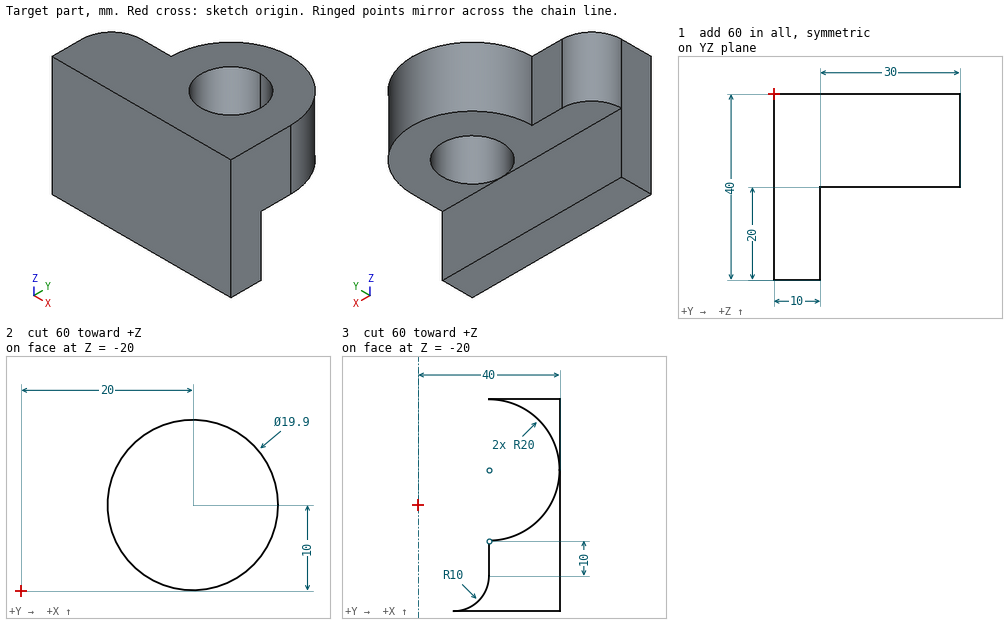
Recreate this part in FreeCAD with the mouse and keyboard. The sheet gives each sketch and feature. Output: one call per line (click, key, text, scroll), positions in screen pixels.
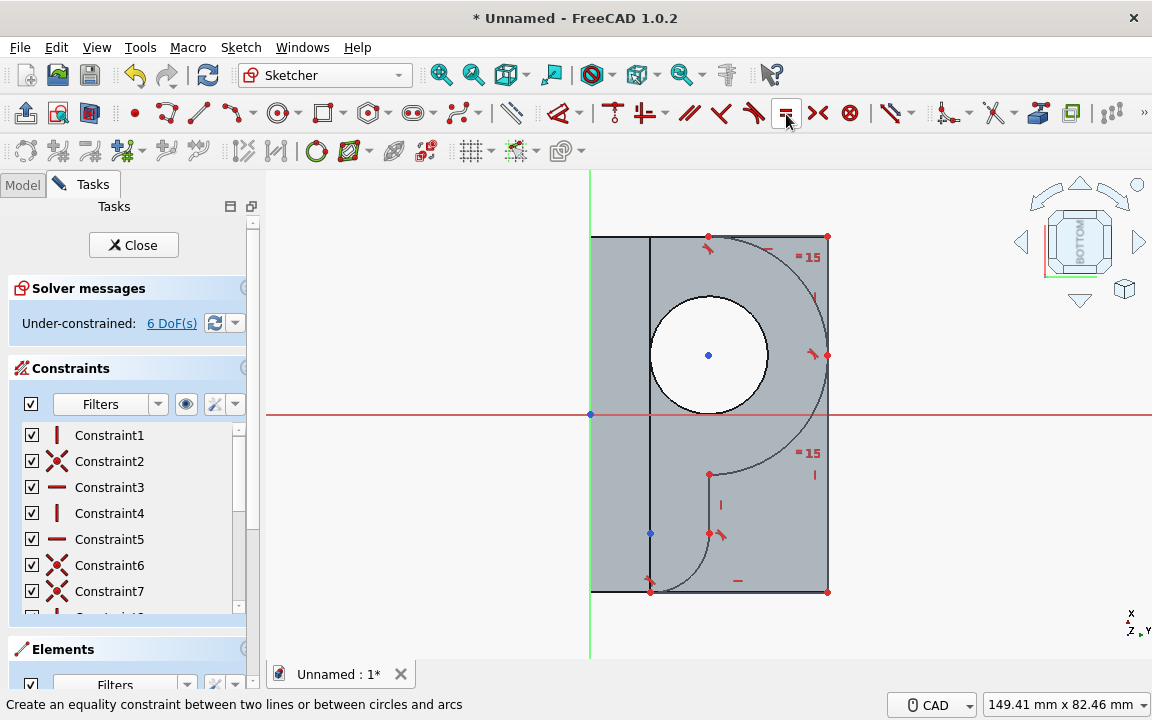
click(709, 356)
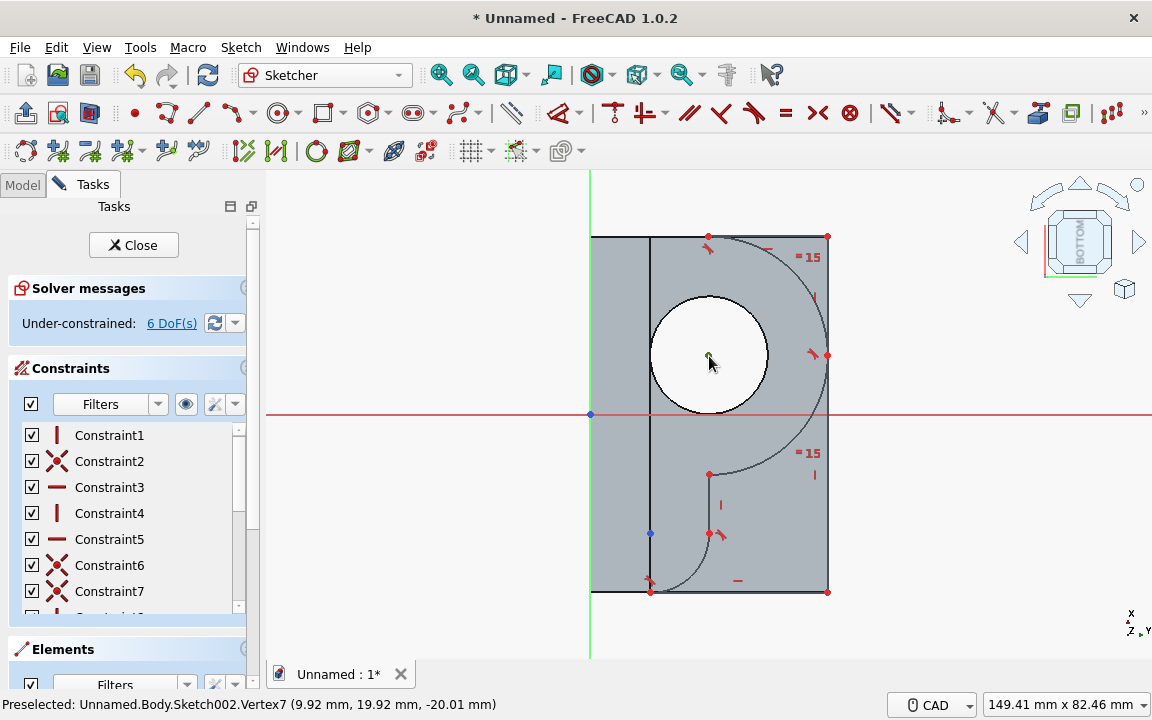
click(709, 475)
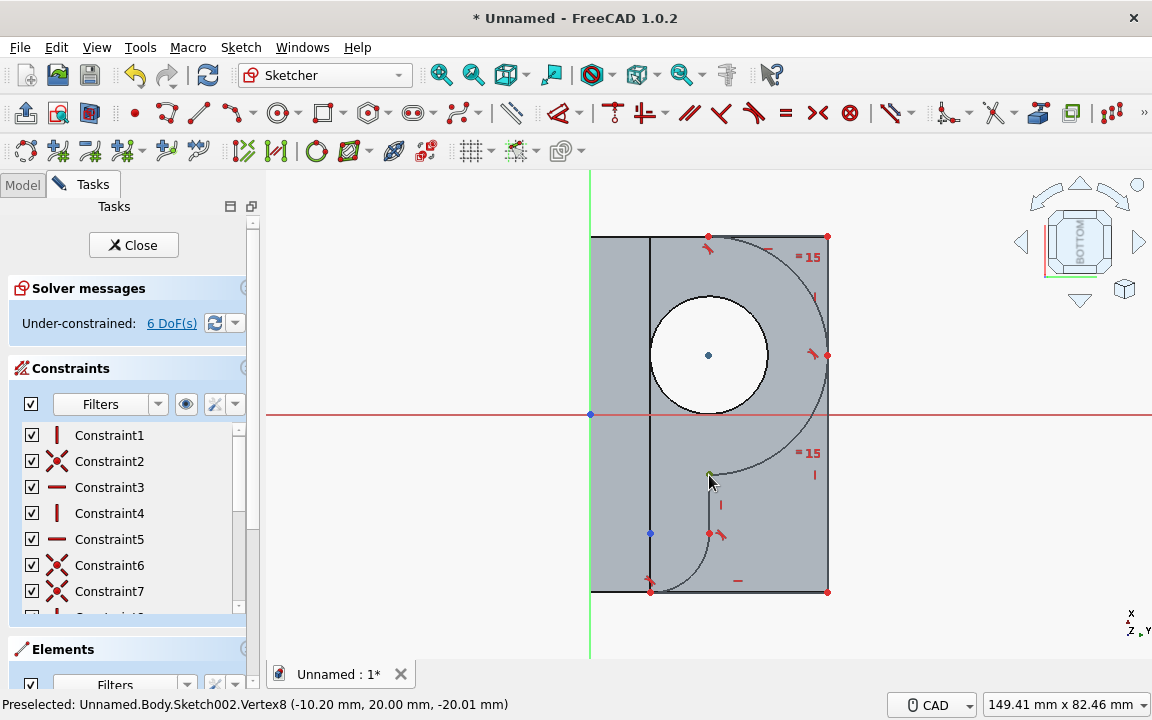
click(344, 414)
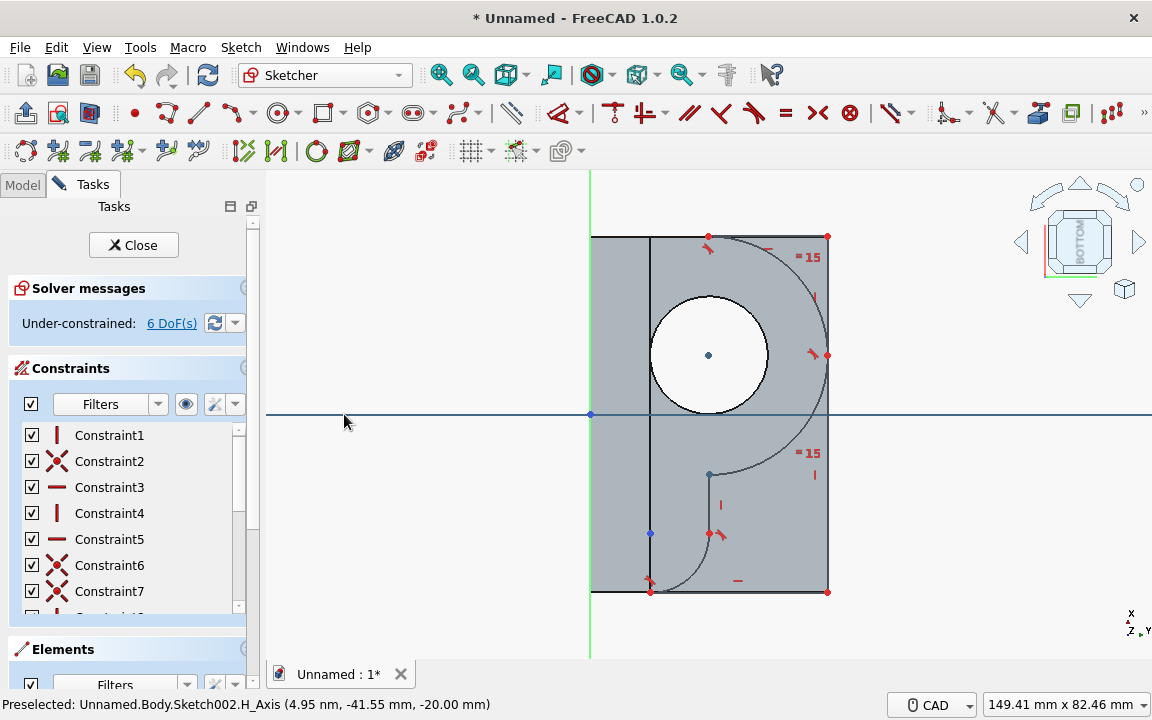
click(818, 114)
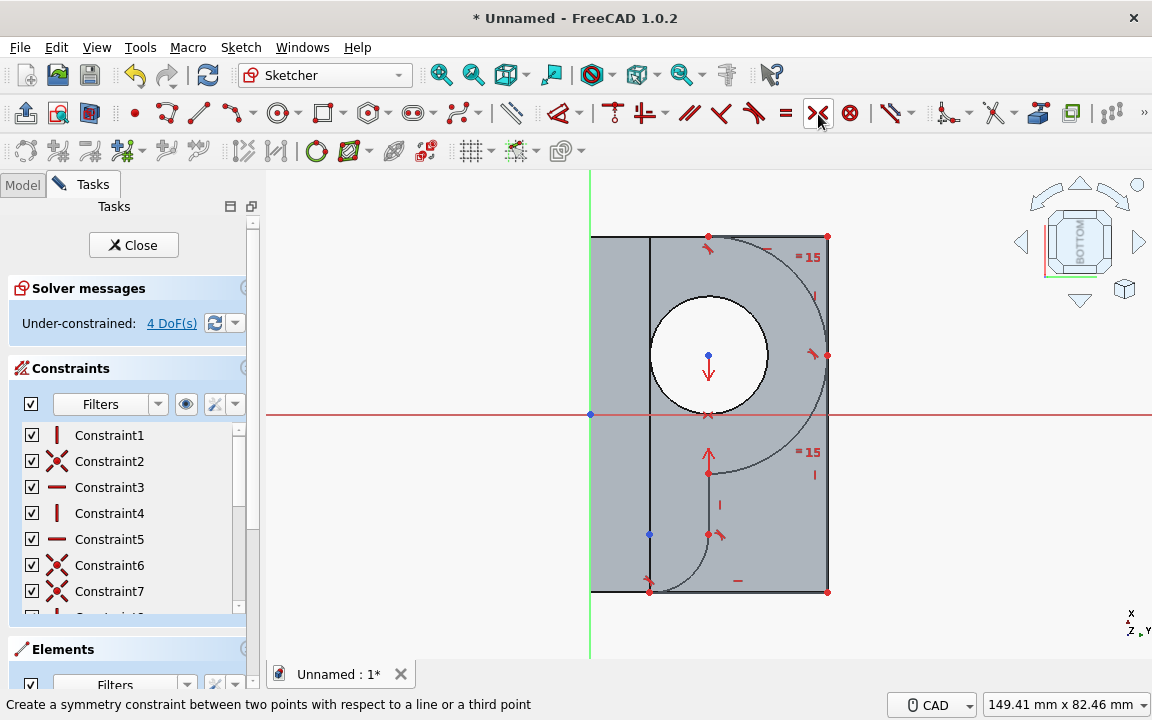
click(558, 114)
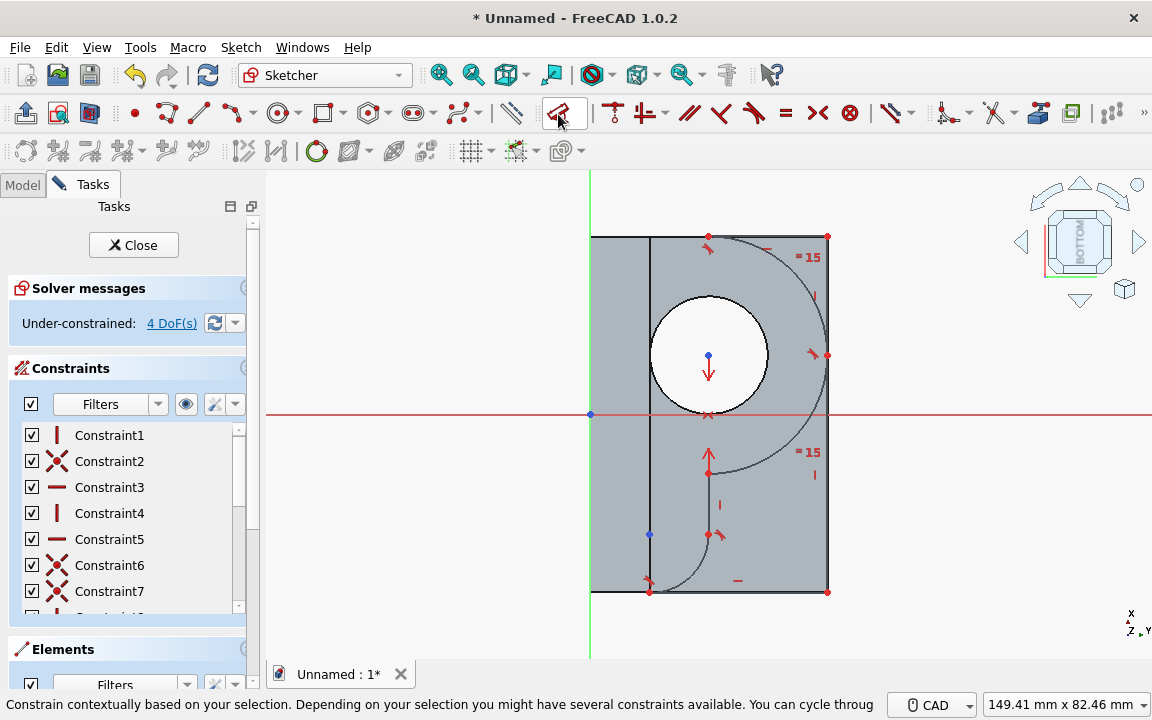
click(814, 301)
click(842, 286)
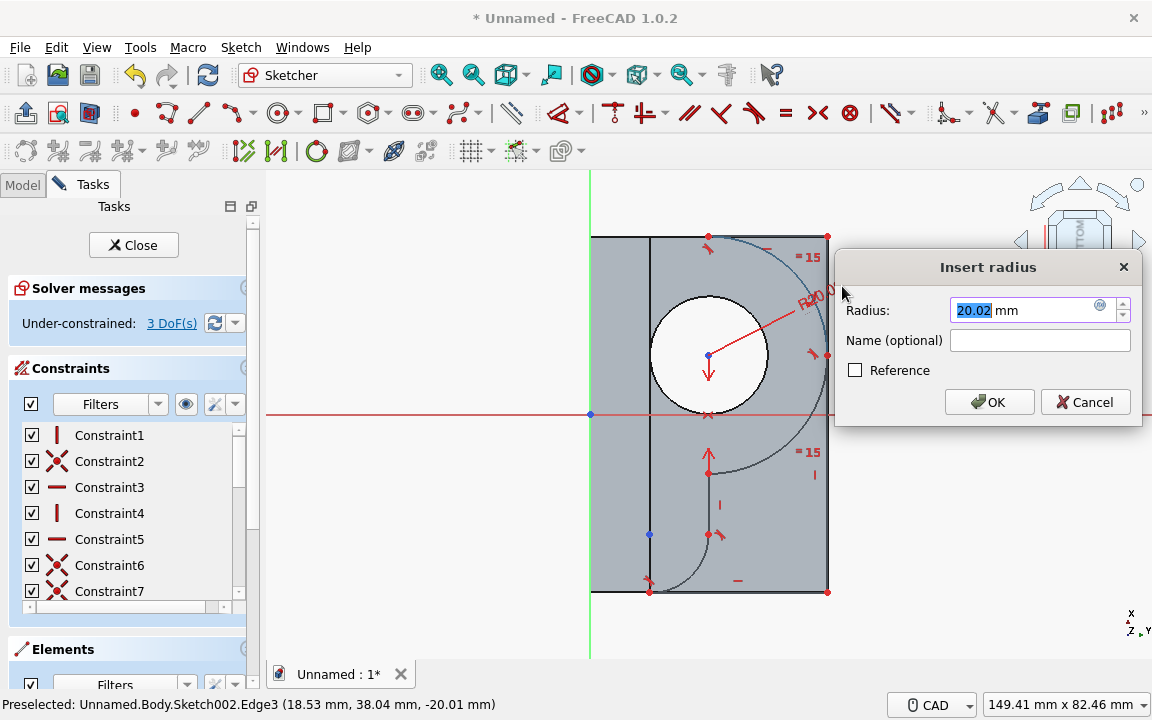
text(20)
key(Return)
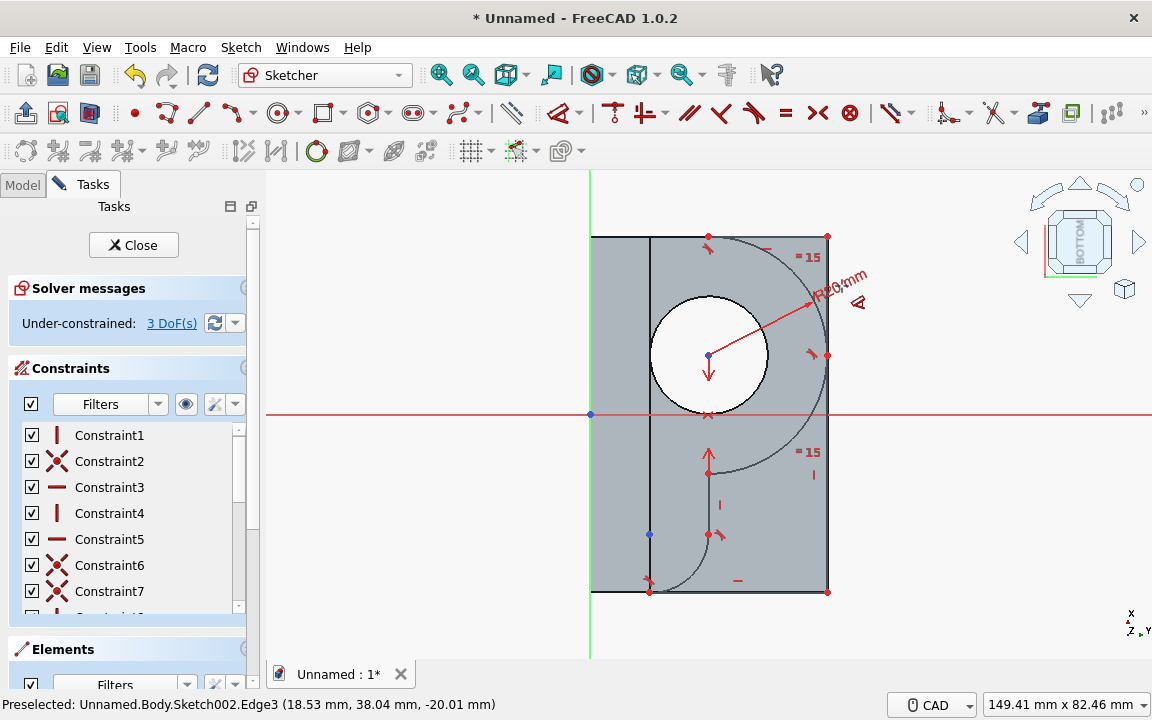
click(702, 561)
click(730, 576)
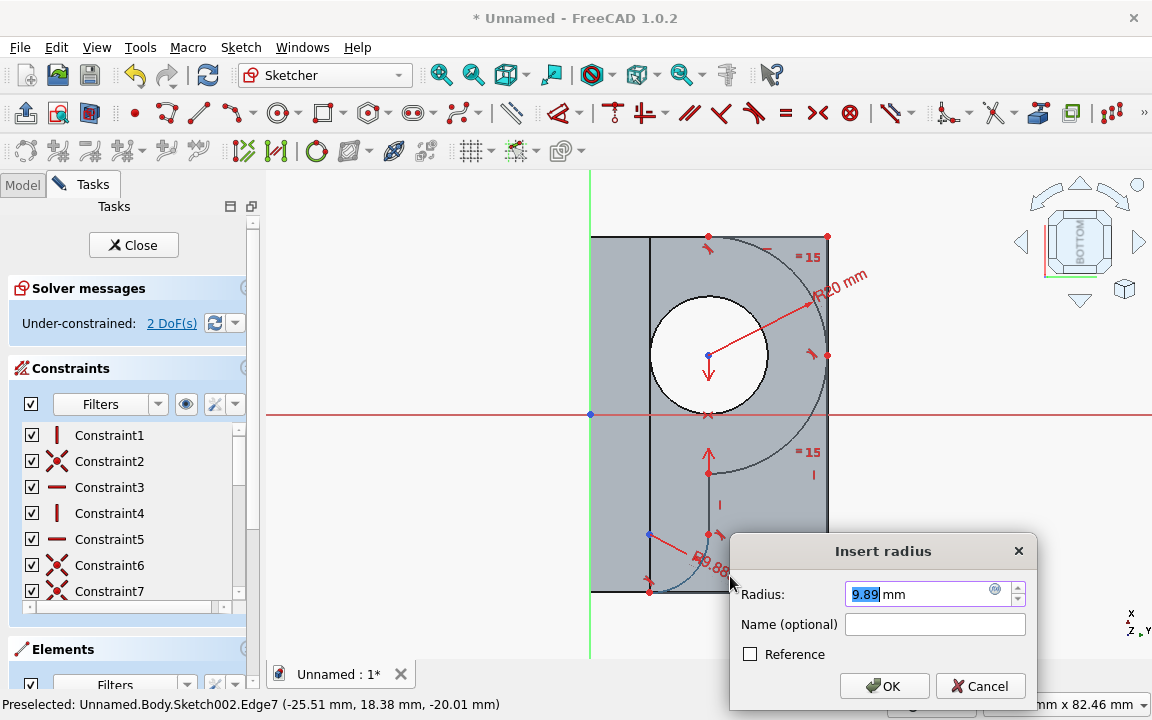
text(10)
key(Return)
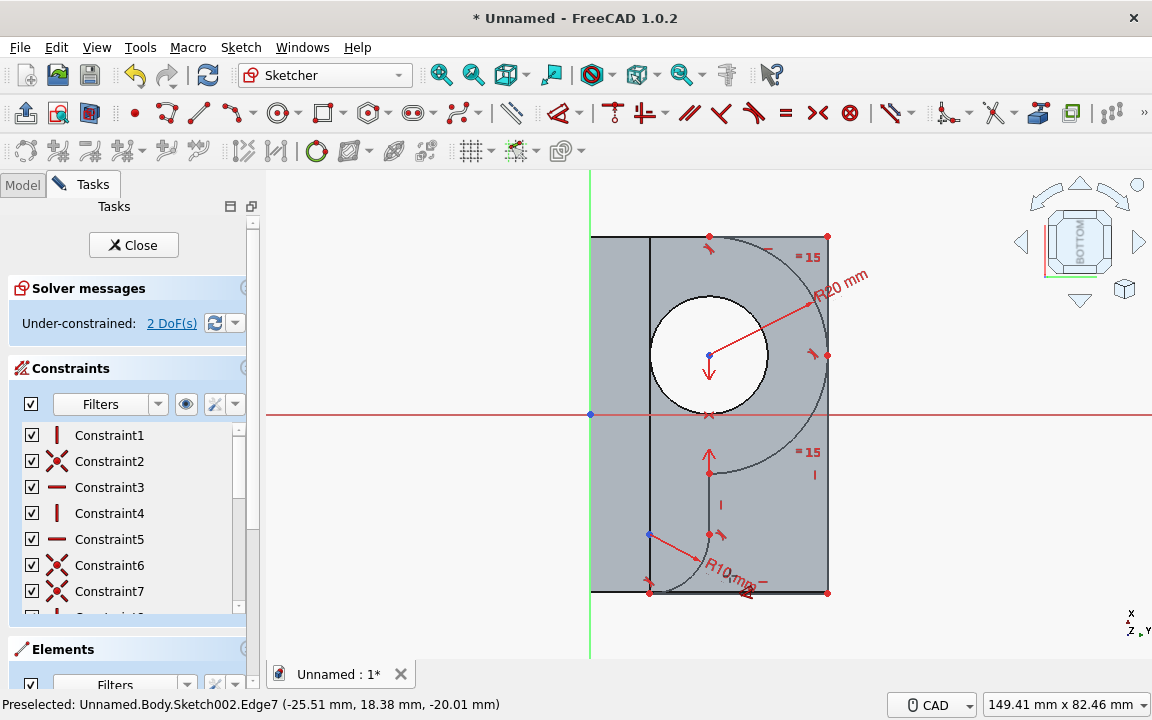
click(709, 492)
click(743, 504)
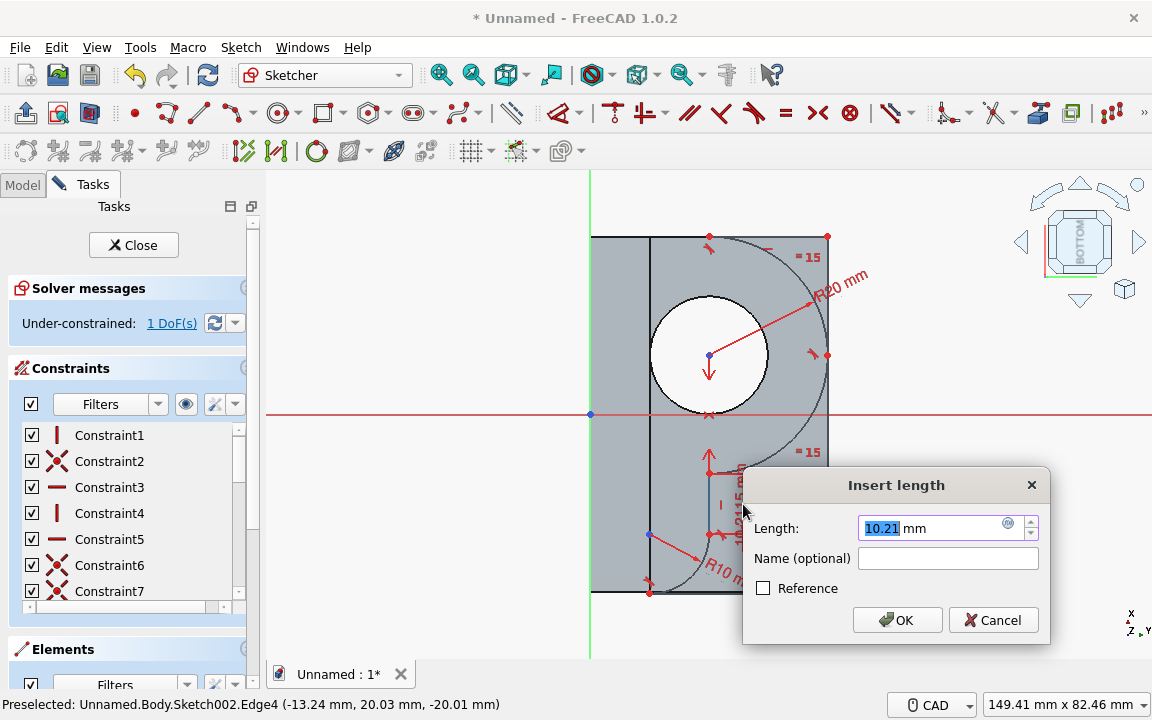
text(10)
key(Return)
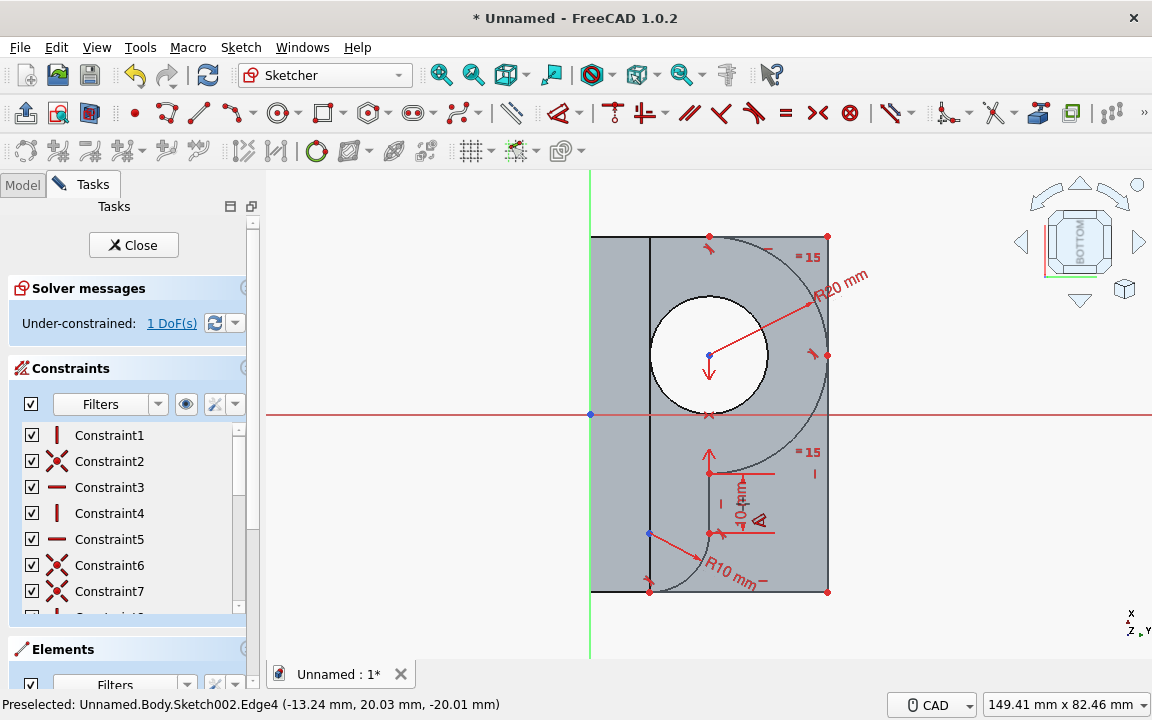
click(828, 355)
click(709, 321)